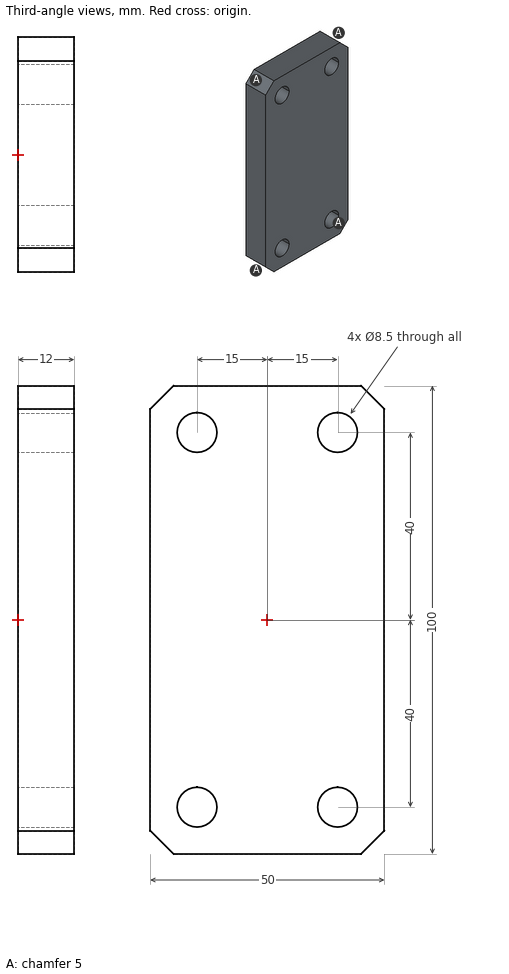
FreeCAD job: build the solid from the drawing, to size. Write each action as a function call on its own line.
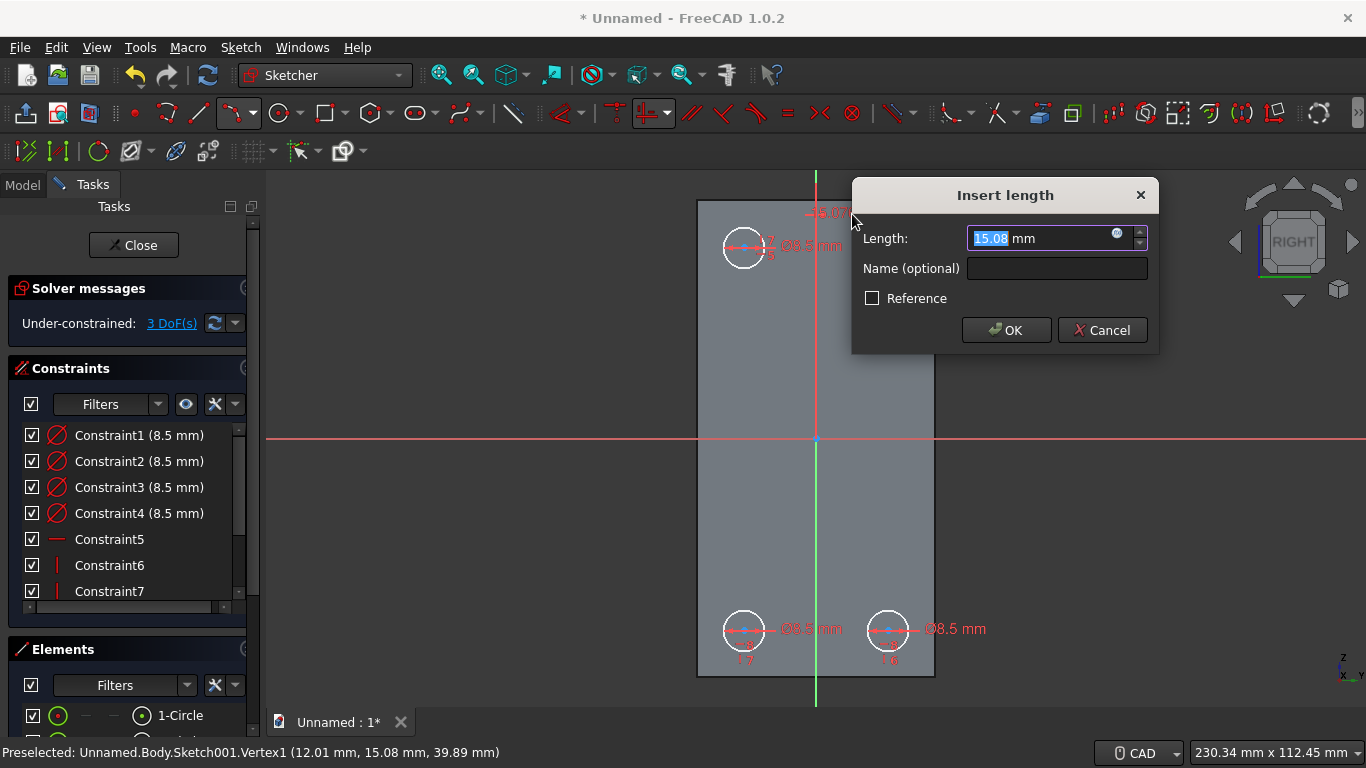
text(15)
key(Return)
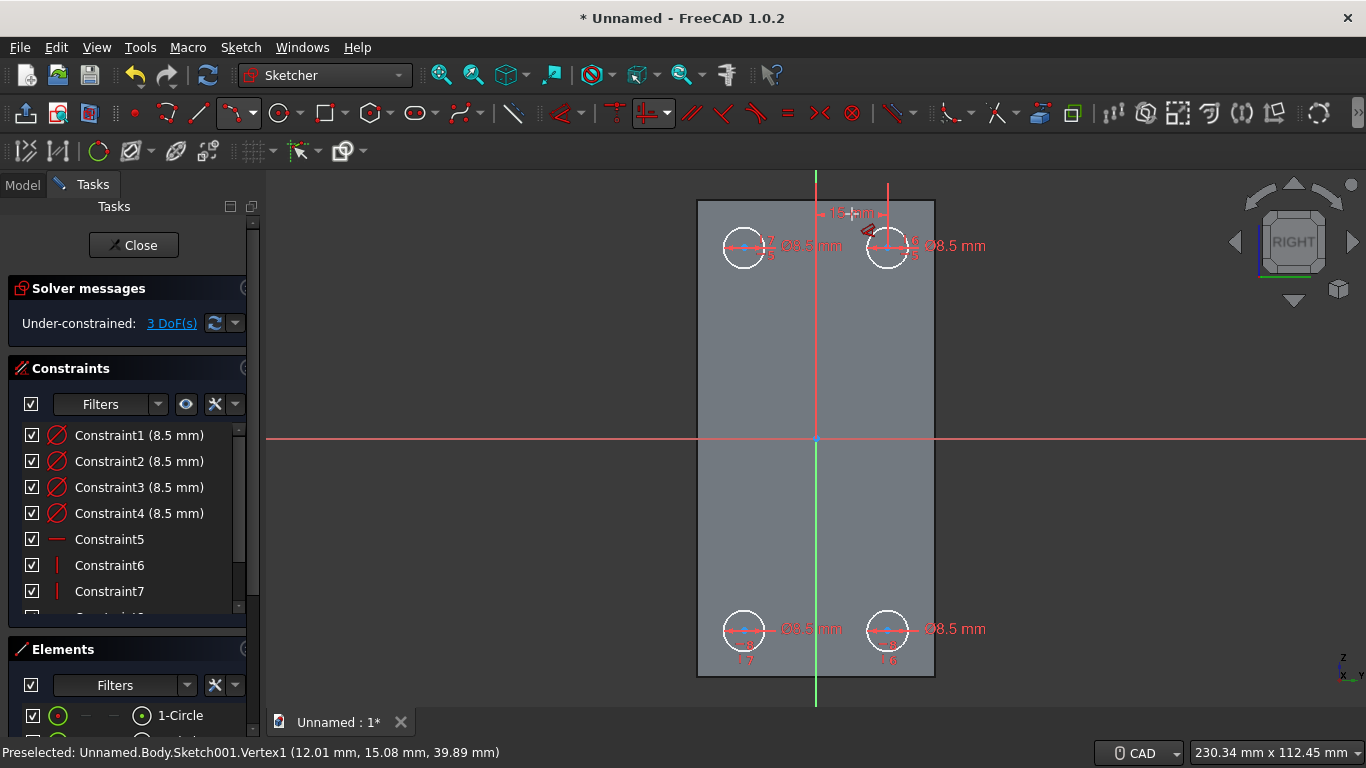
click(888, 248)
click(922, 343)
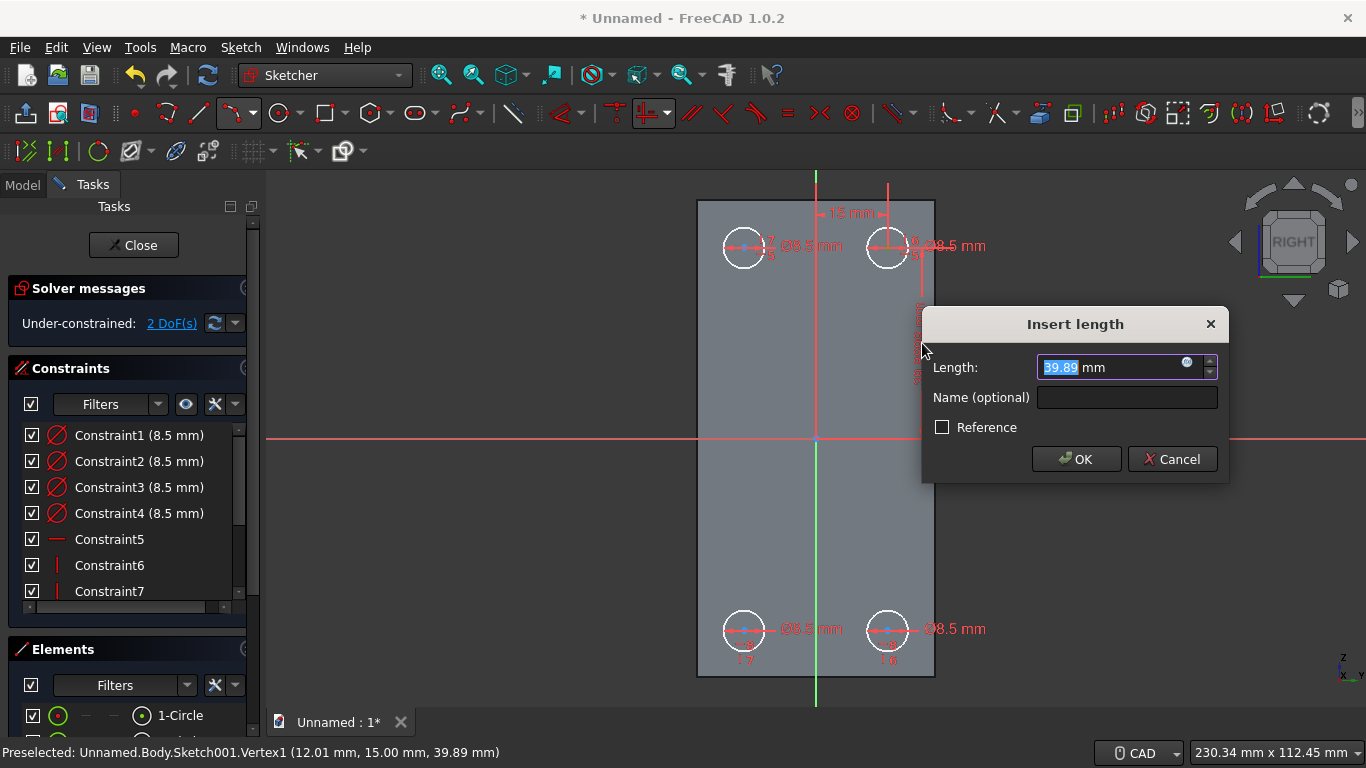
text(40)
key(Return)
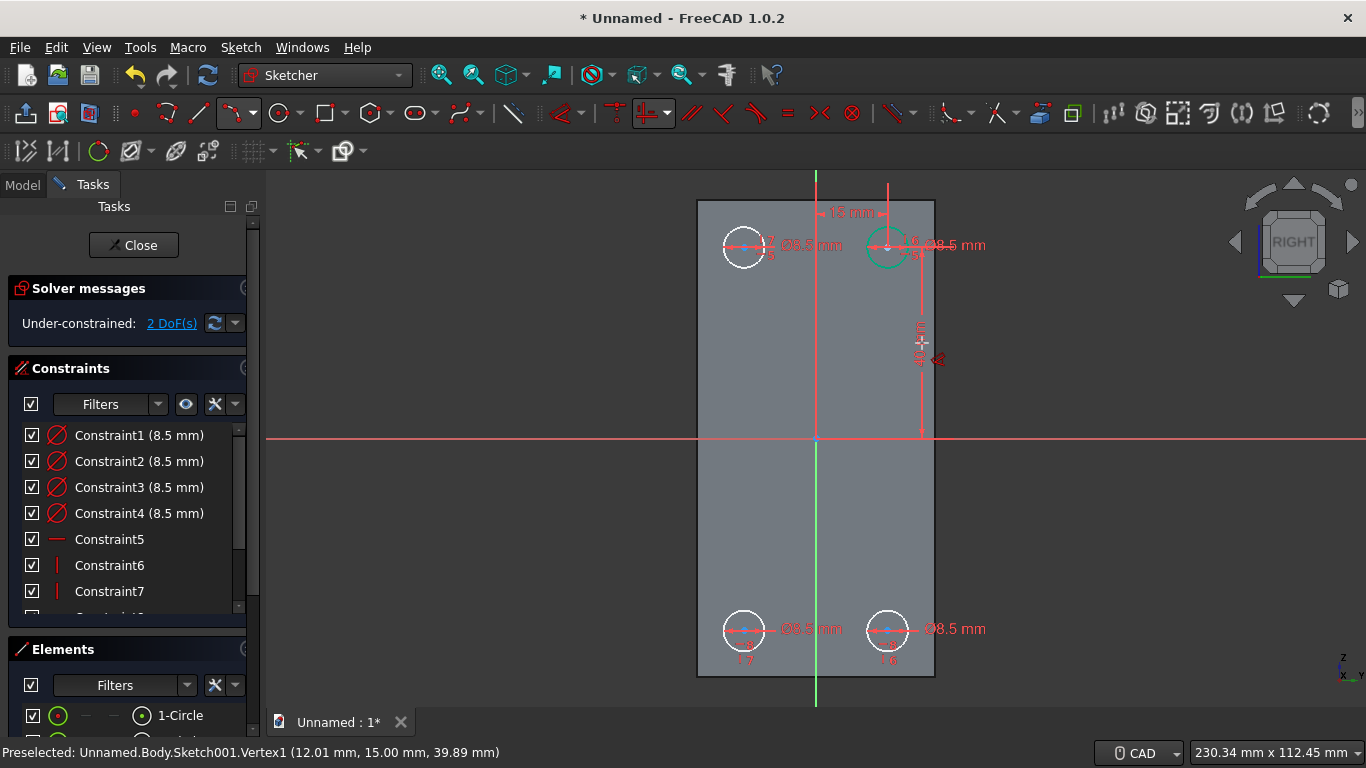
click(744, 247)
click(780, 213)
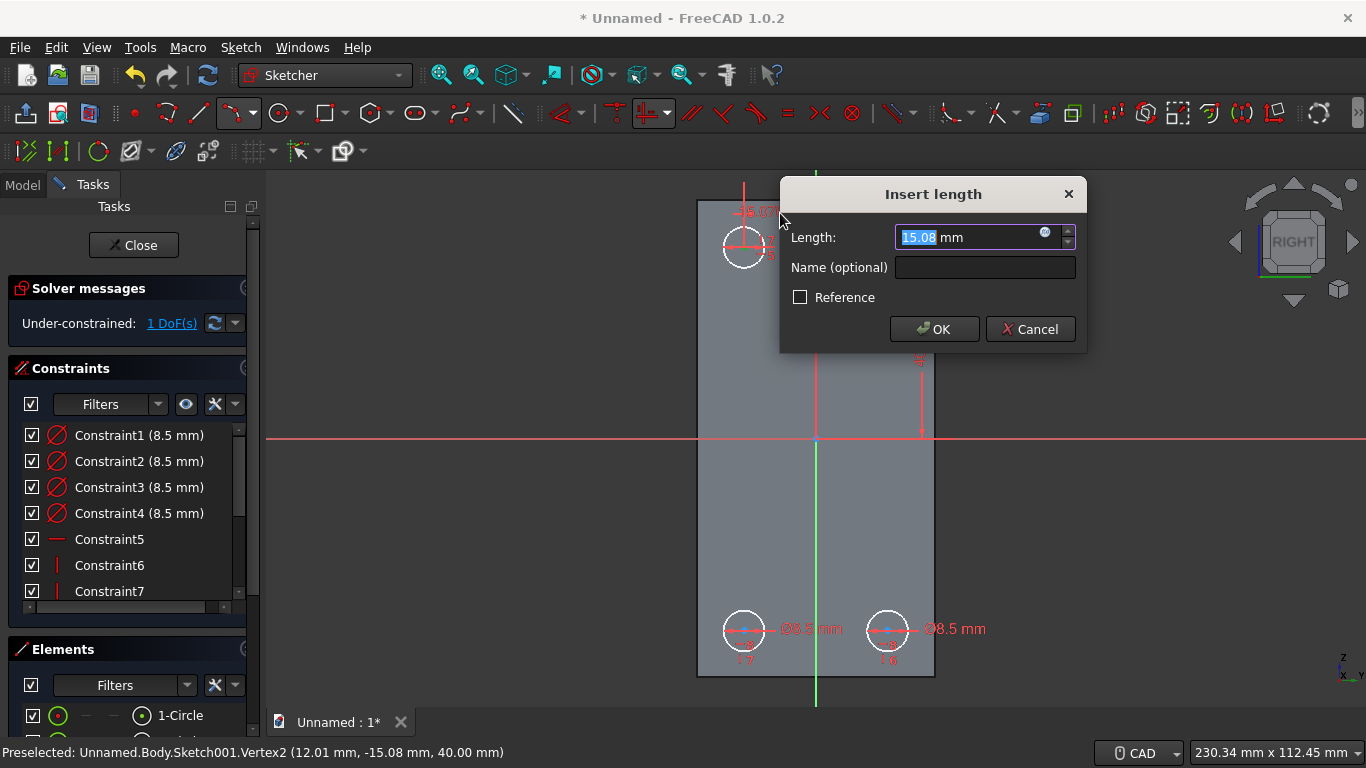
text(15)
key(Return)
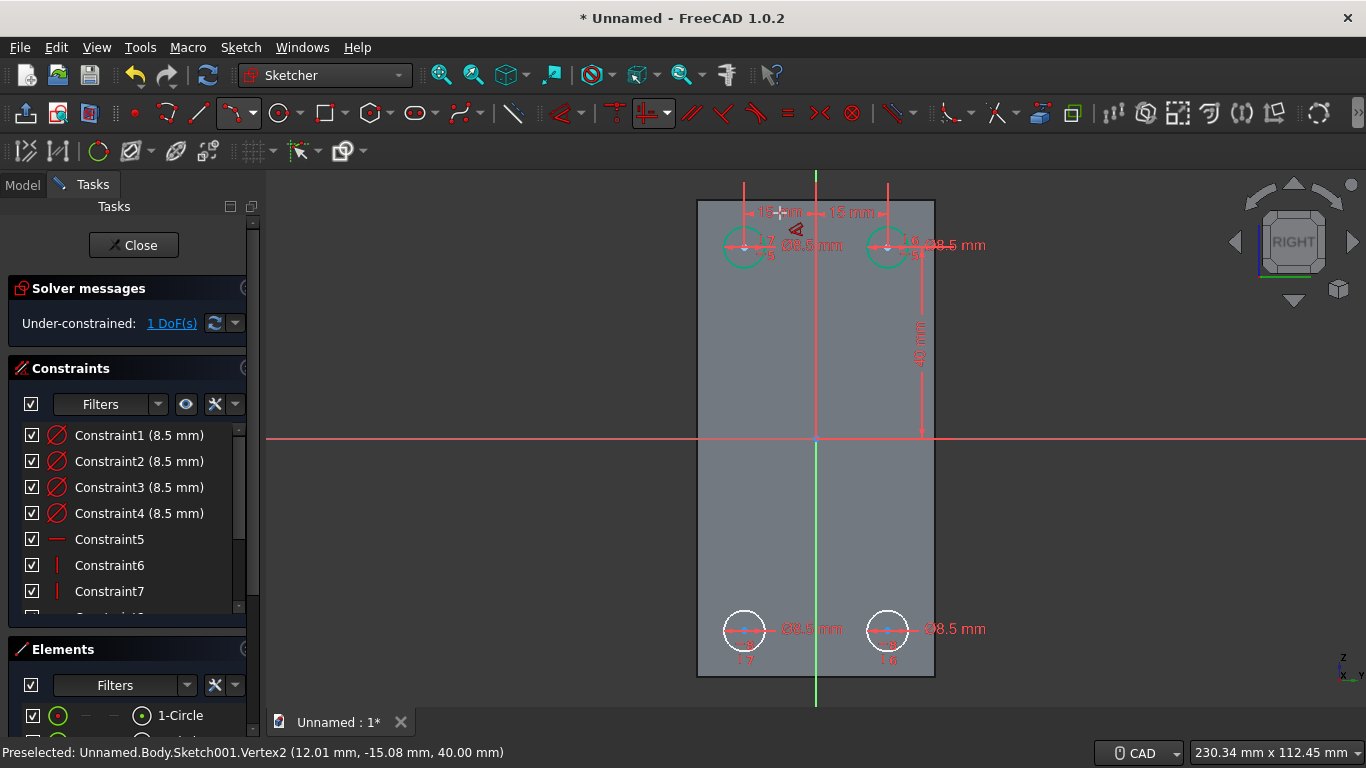
click(888, 631)
click(922, 535)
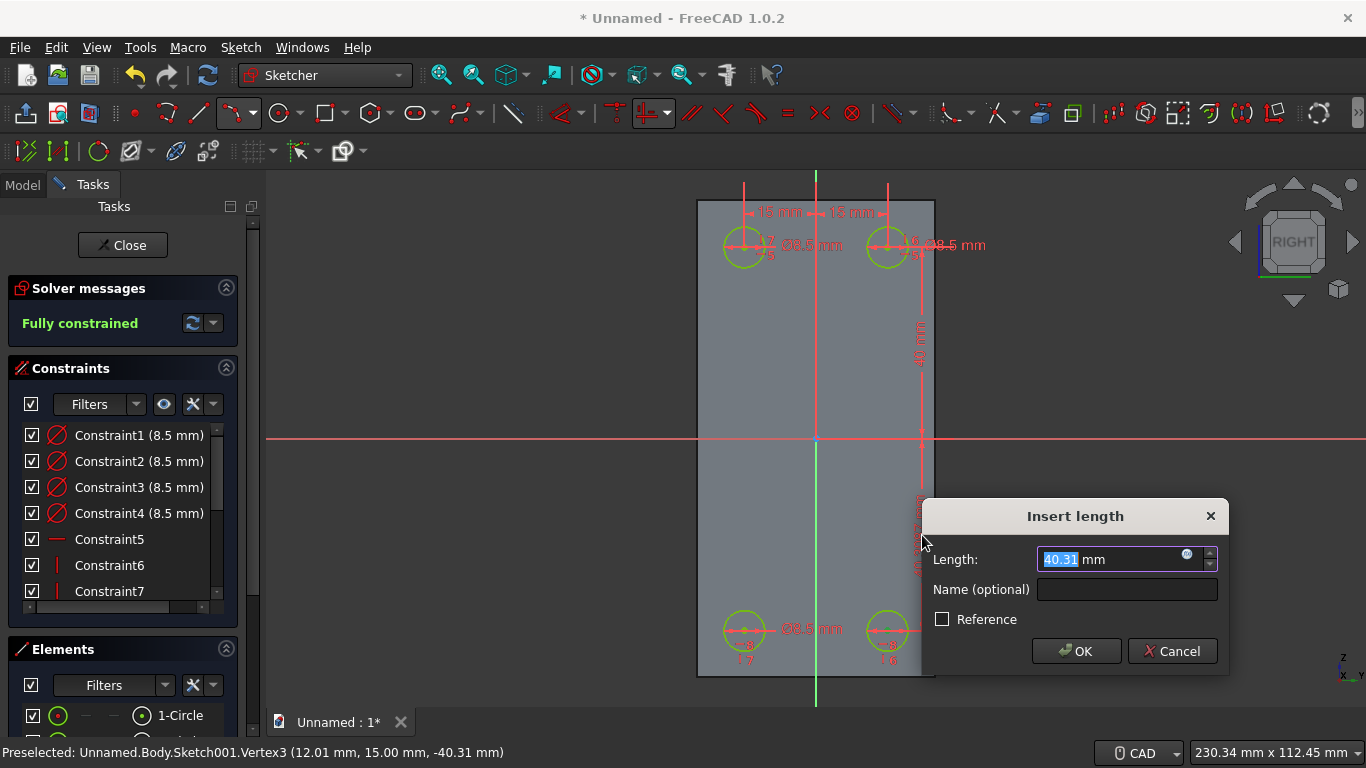
text(40)
key(Return)
key(Escape)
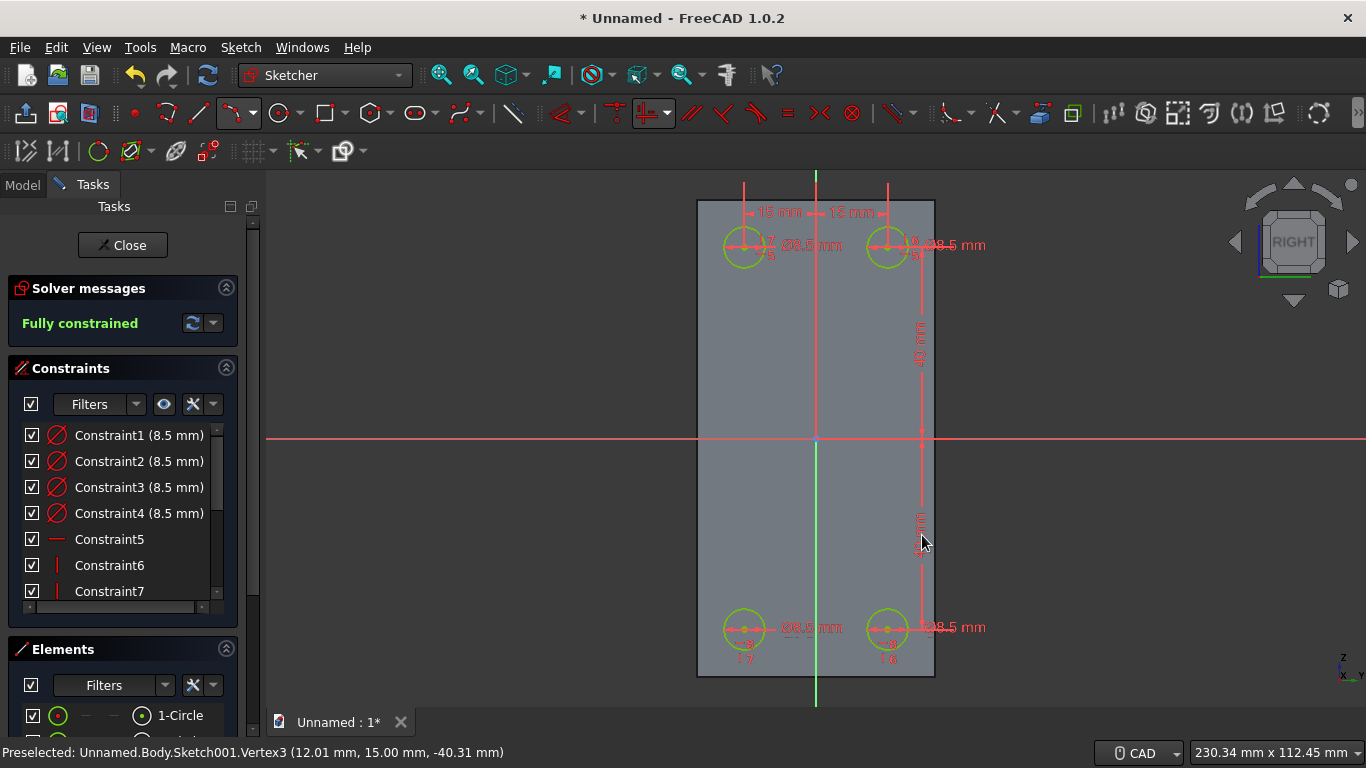
click(123, 245)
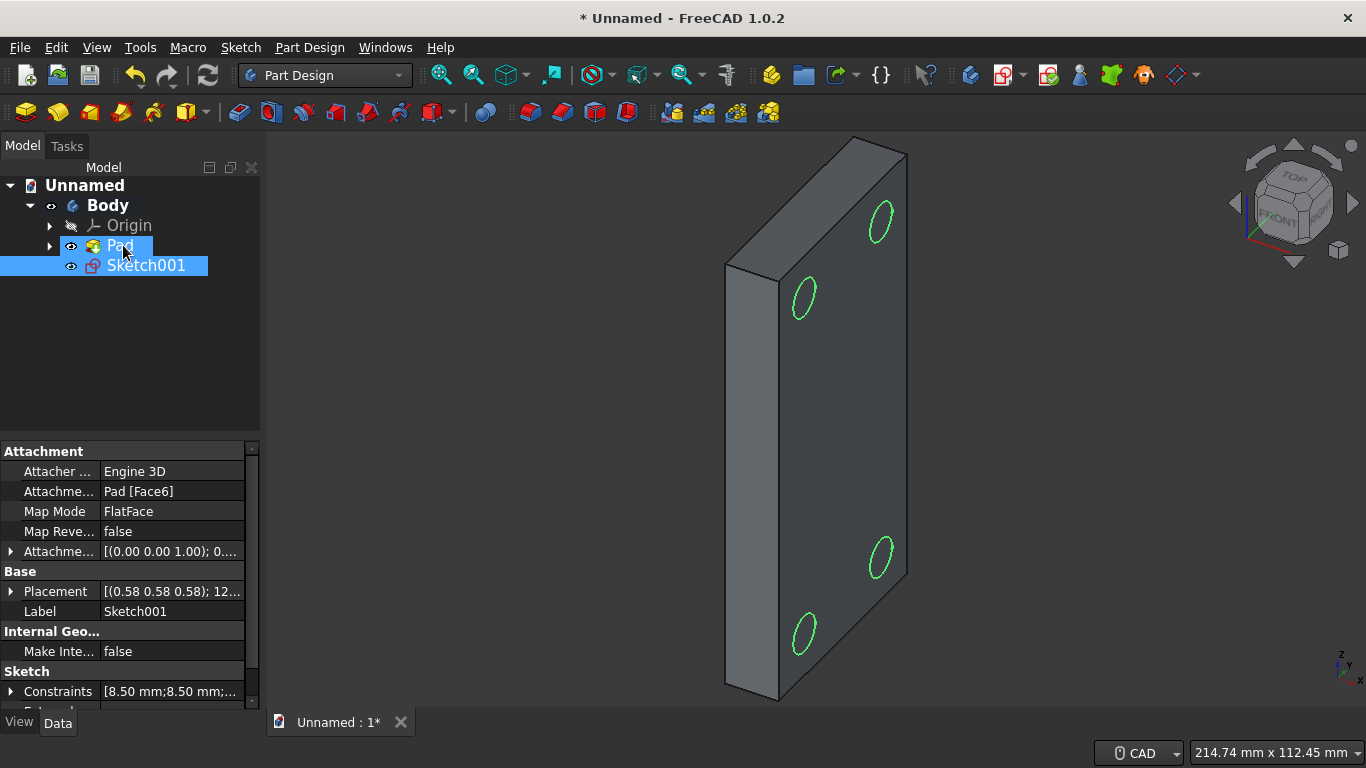
click(272, 112)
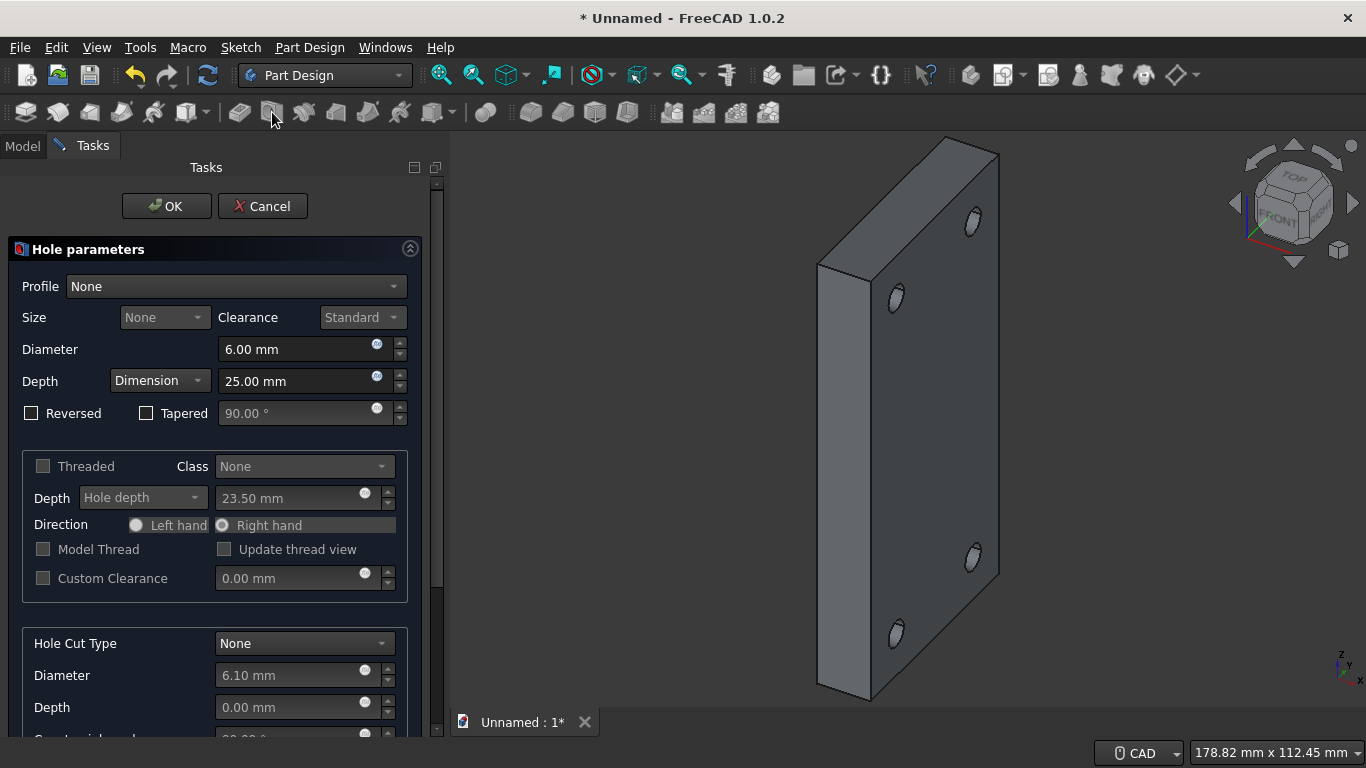
triple_click(305, 349)